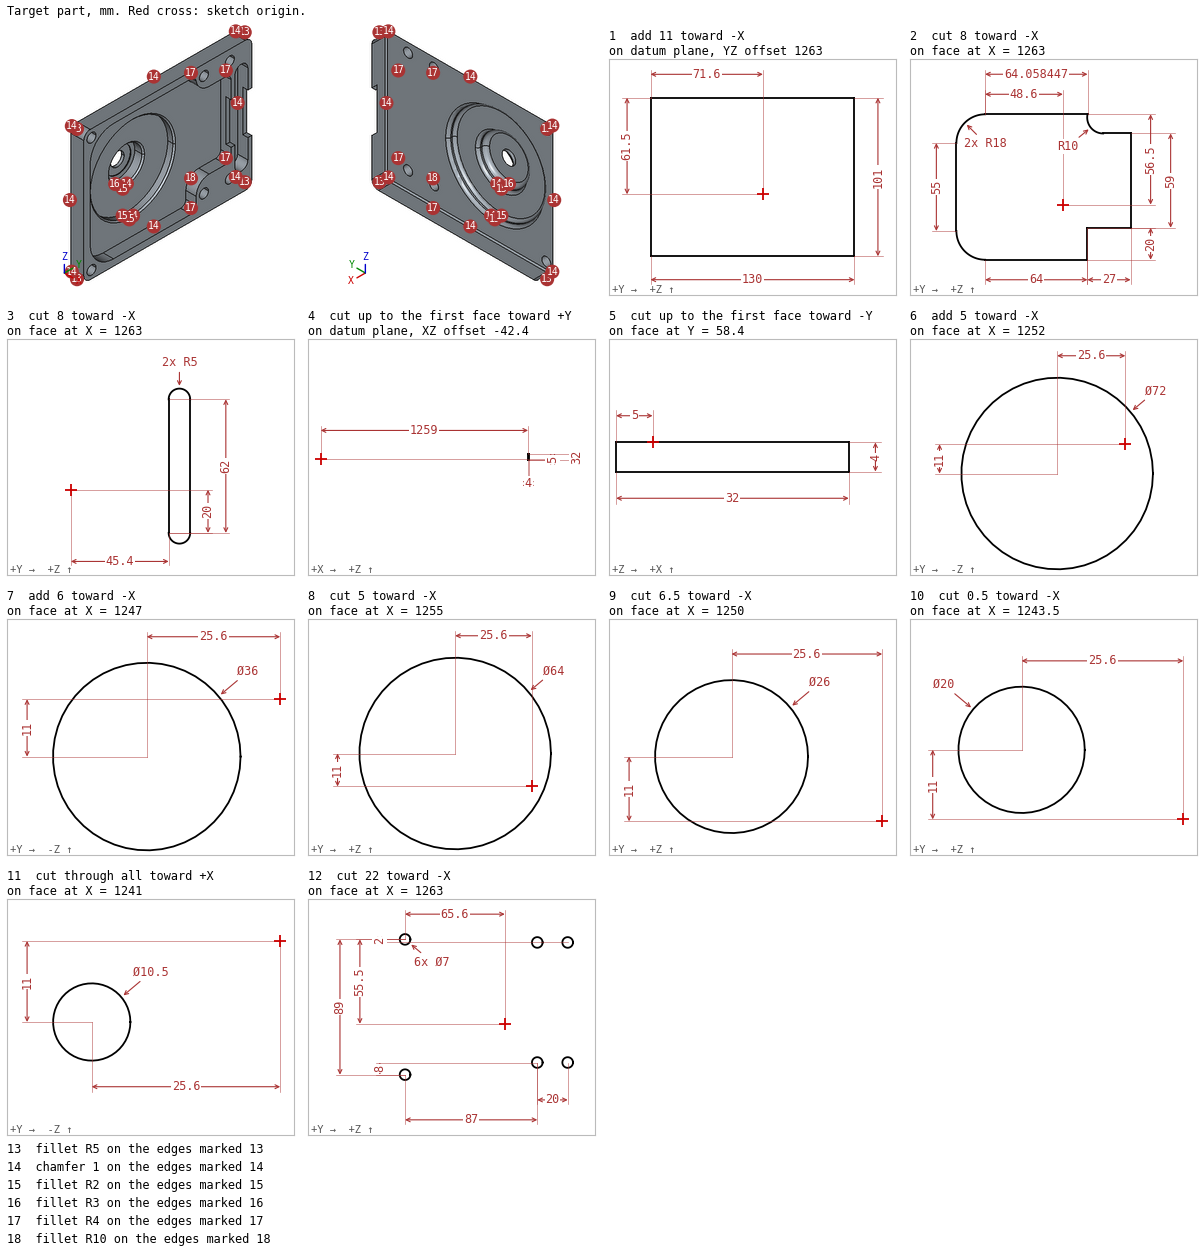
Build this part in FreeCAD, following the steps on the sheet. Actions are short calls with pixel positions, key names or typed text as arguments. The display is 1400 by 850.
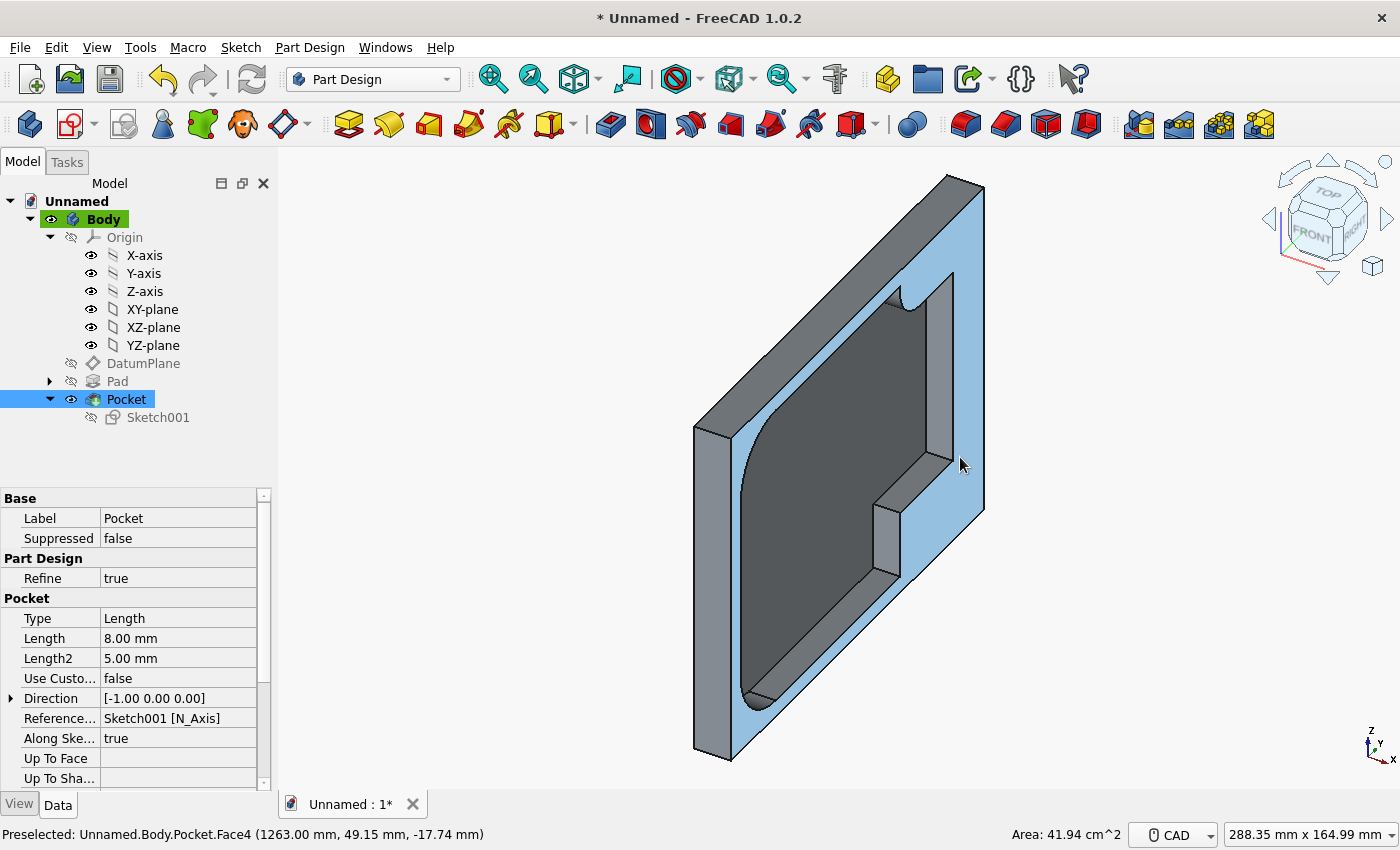
click(70, 124)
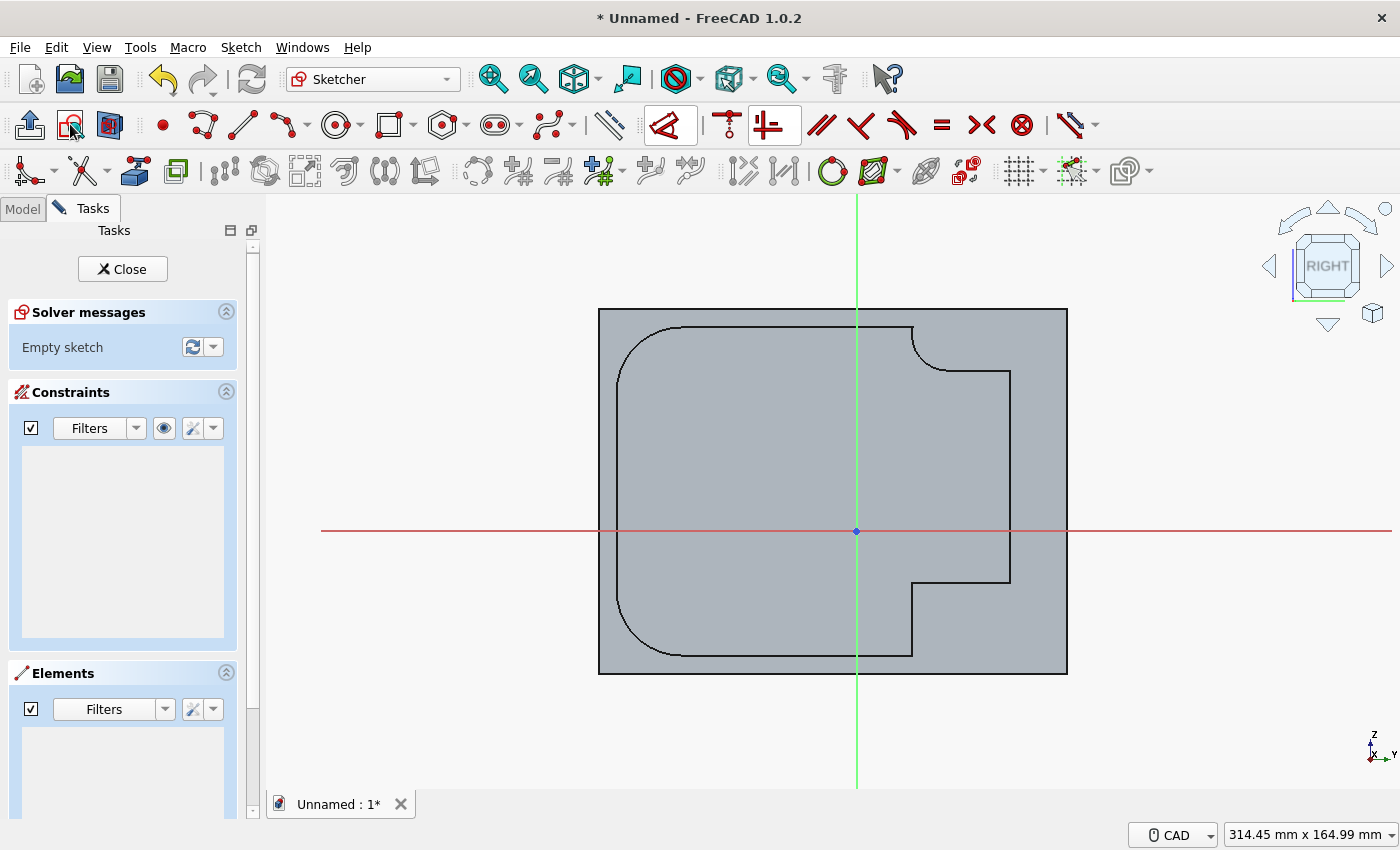
scroll(1235, 492, up, 2)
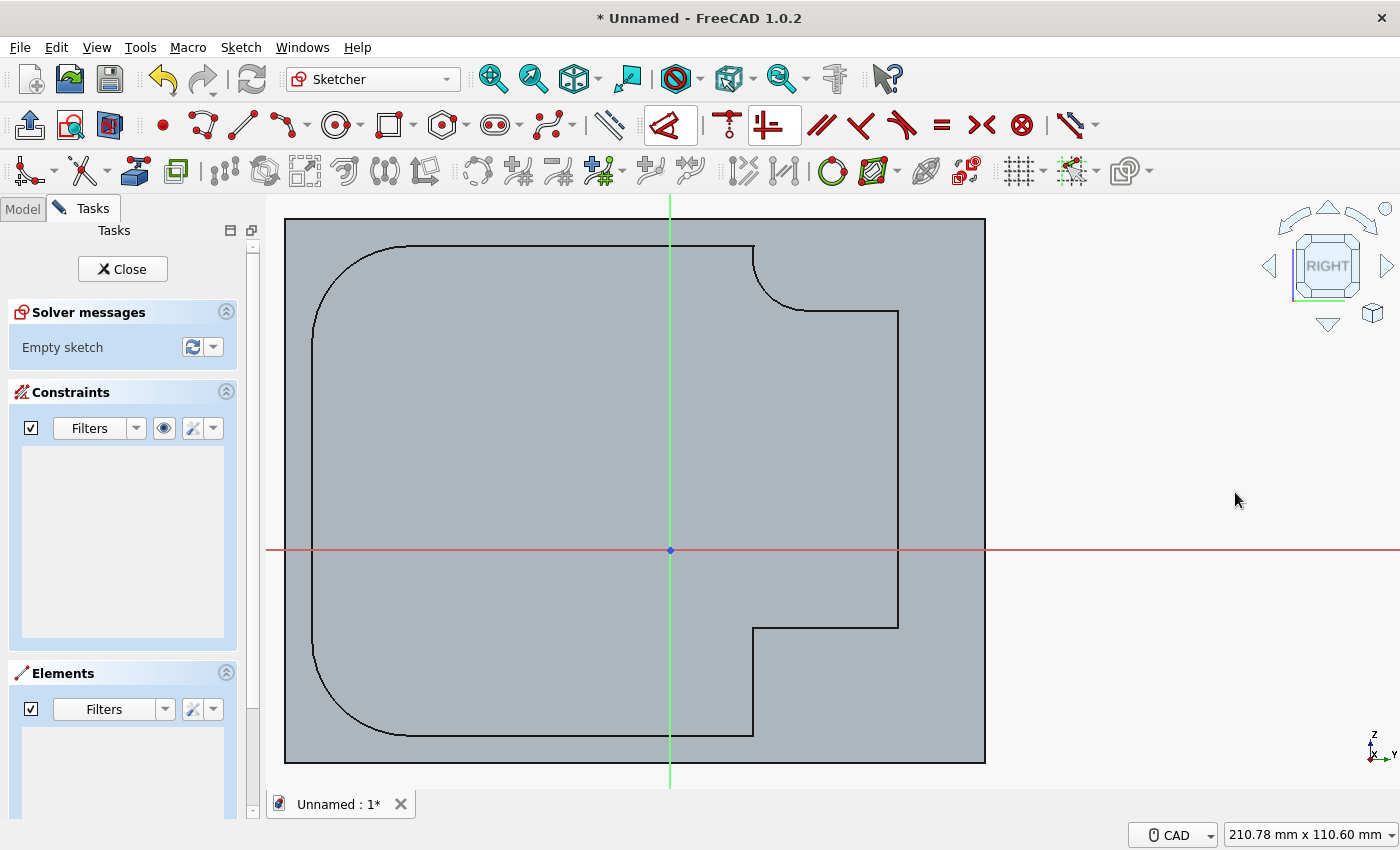
click(496, 126)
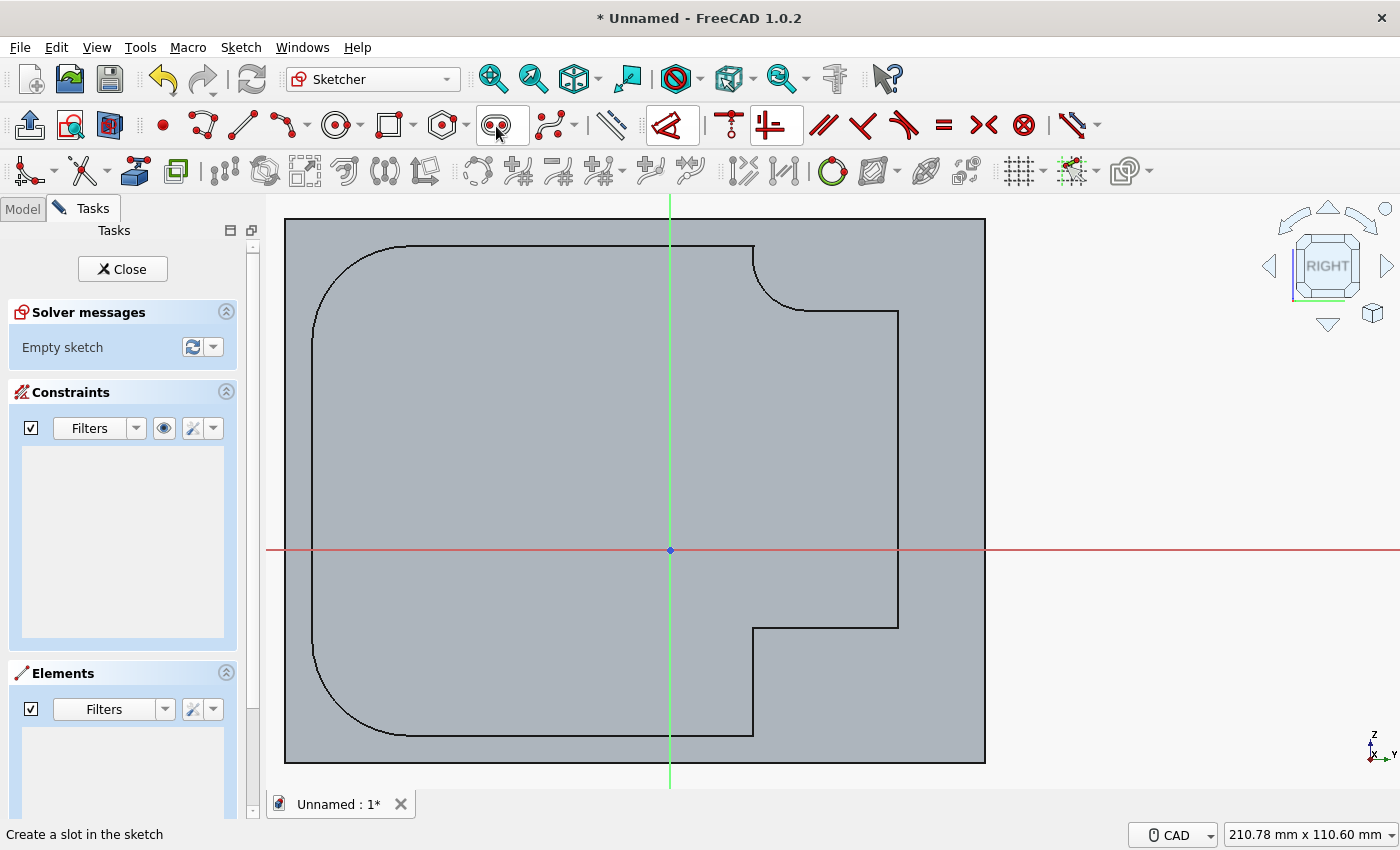
click(942, 658)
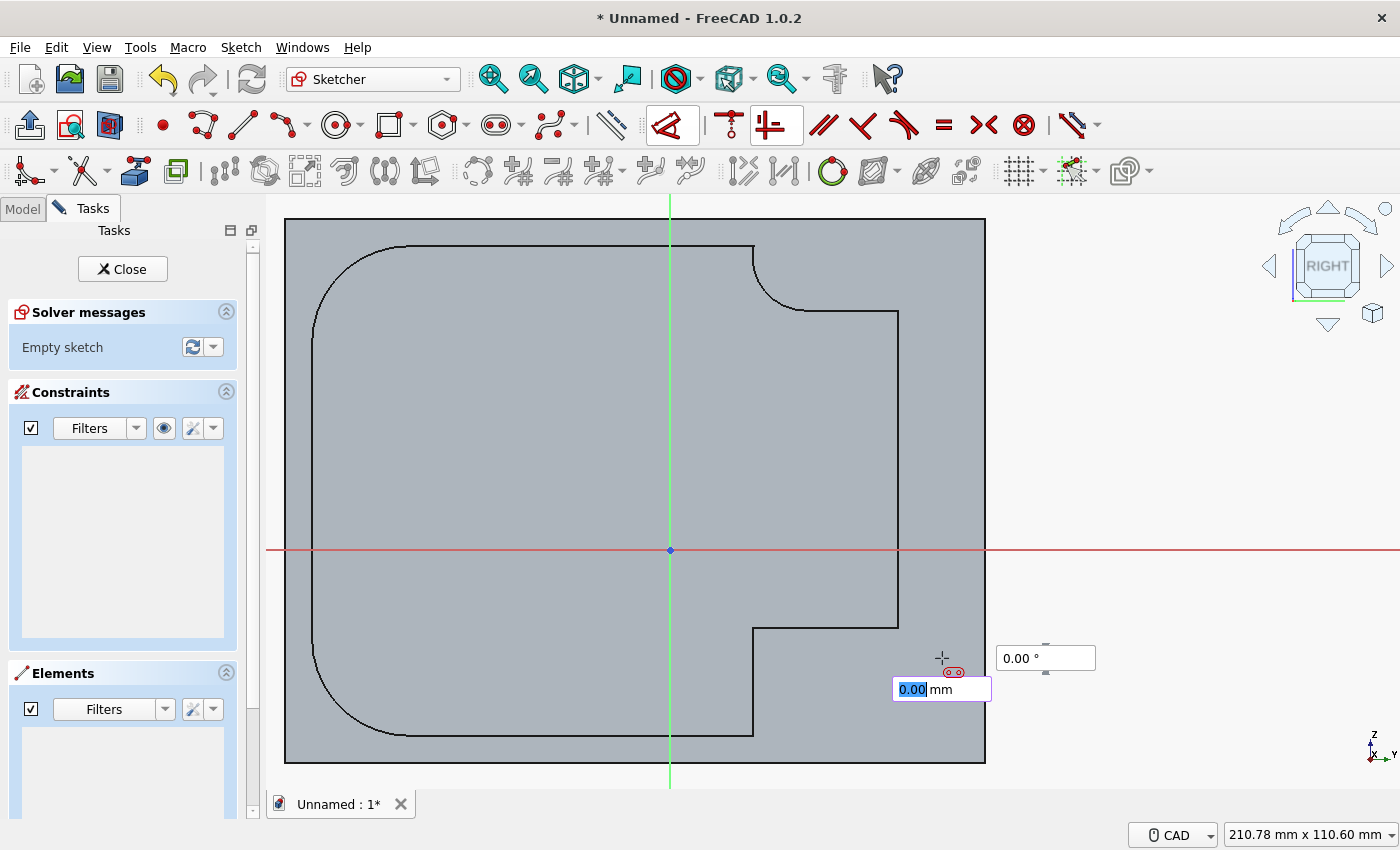
click(942, 324)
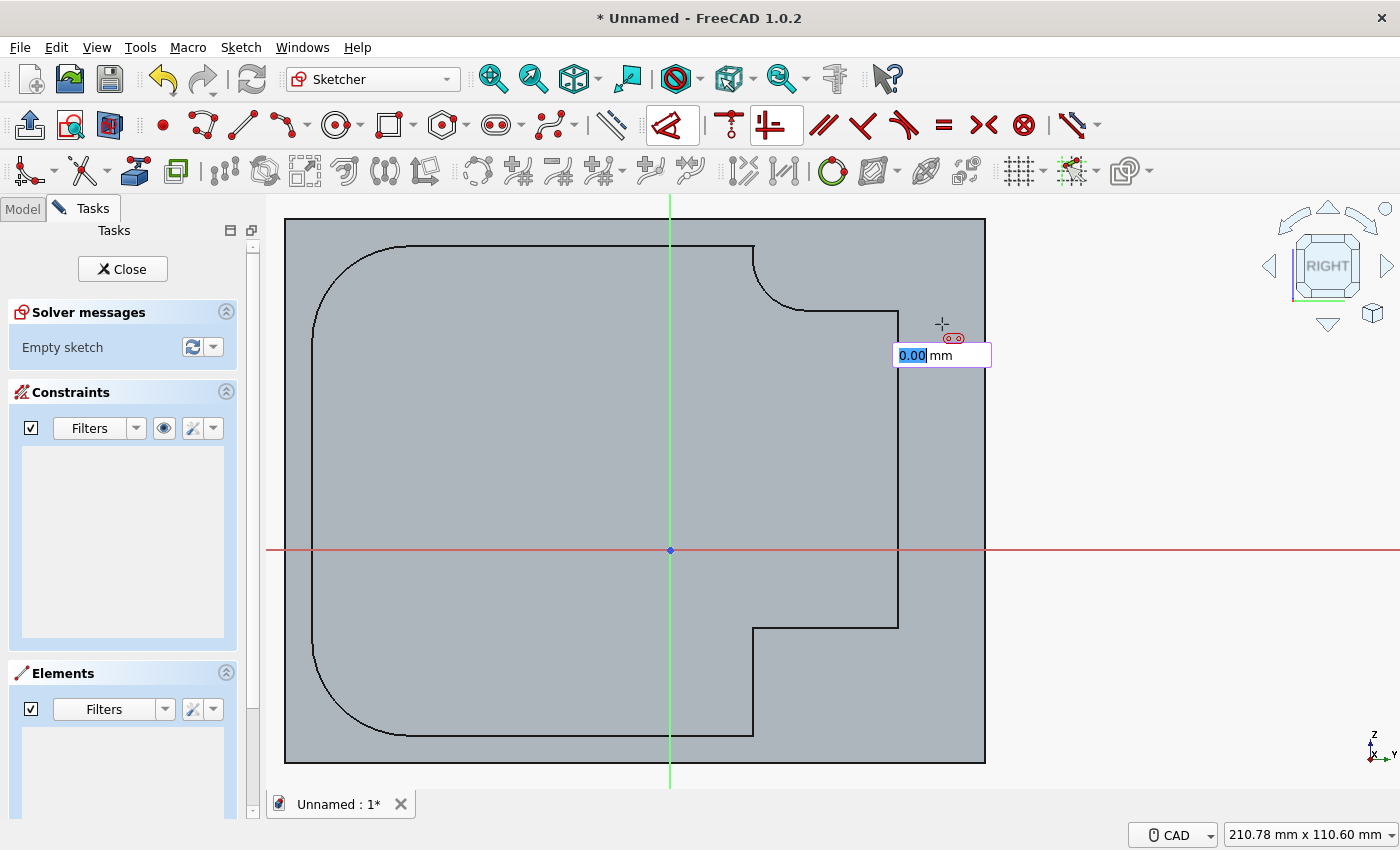
click(968, 491)
key(Escape)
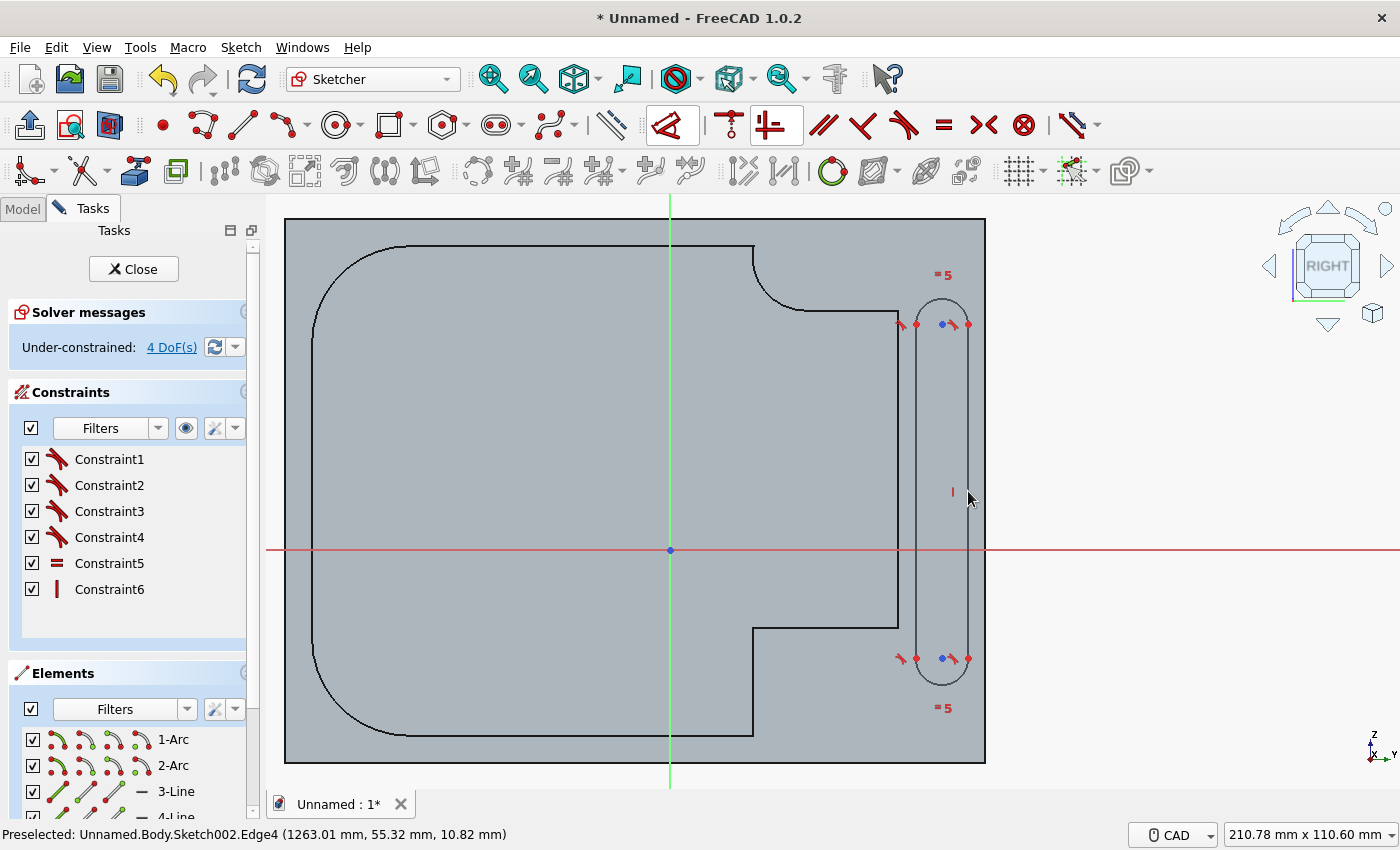
scroll(927, 680, up, 2)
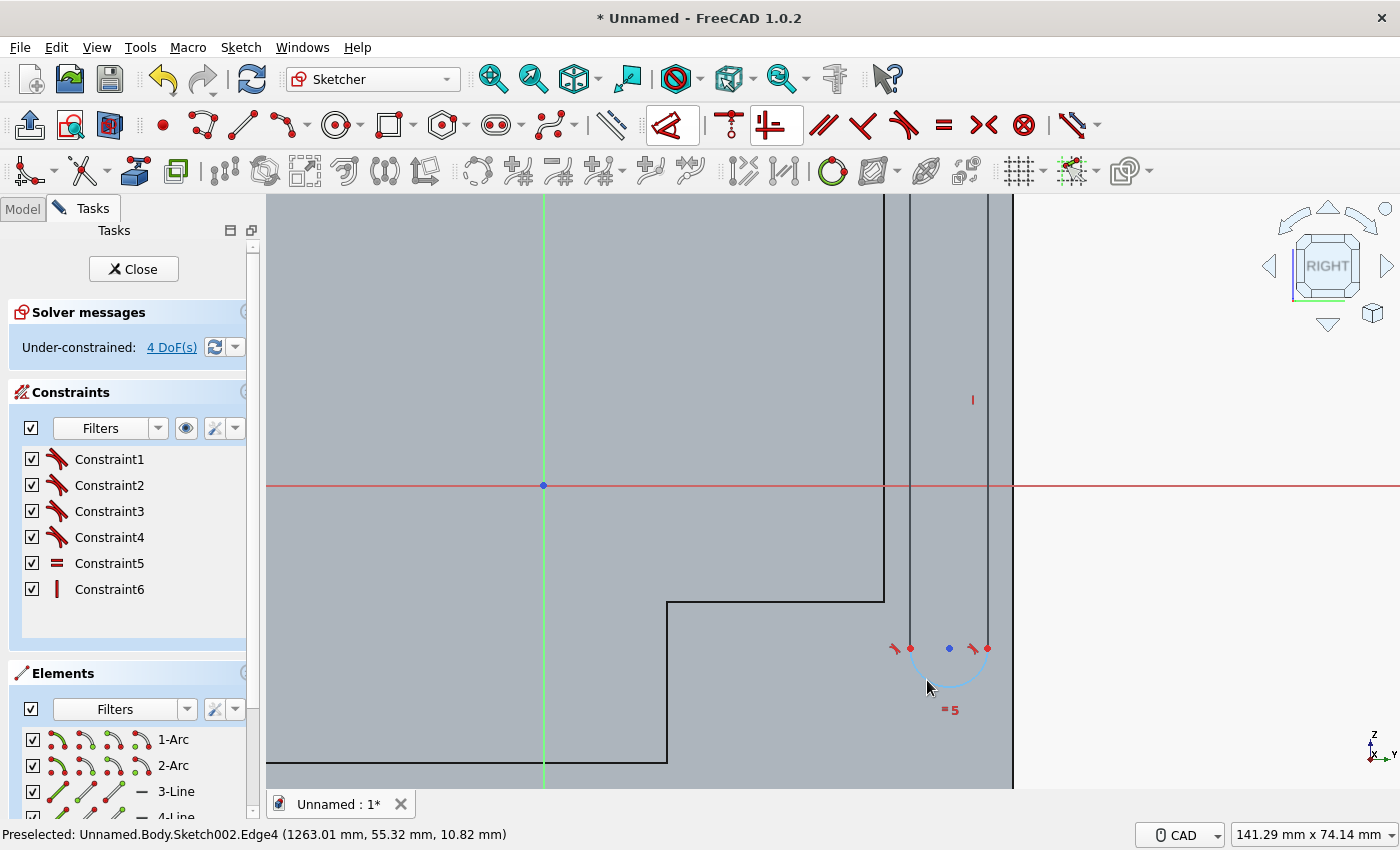
click(926, 680)